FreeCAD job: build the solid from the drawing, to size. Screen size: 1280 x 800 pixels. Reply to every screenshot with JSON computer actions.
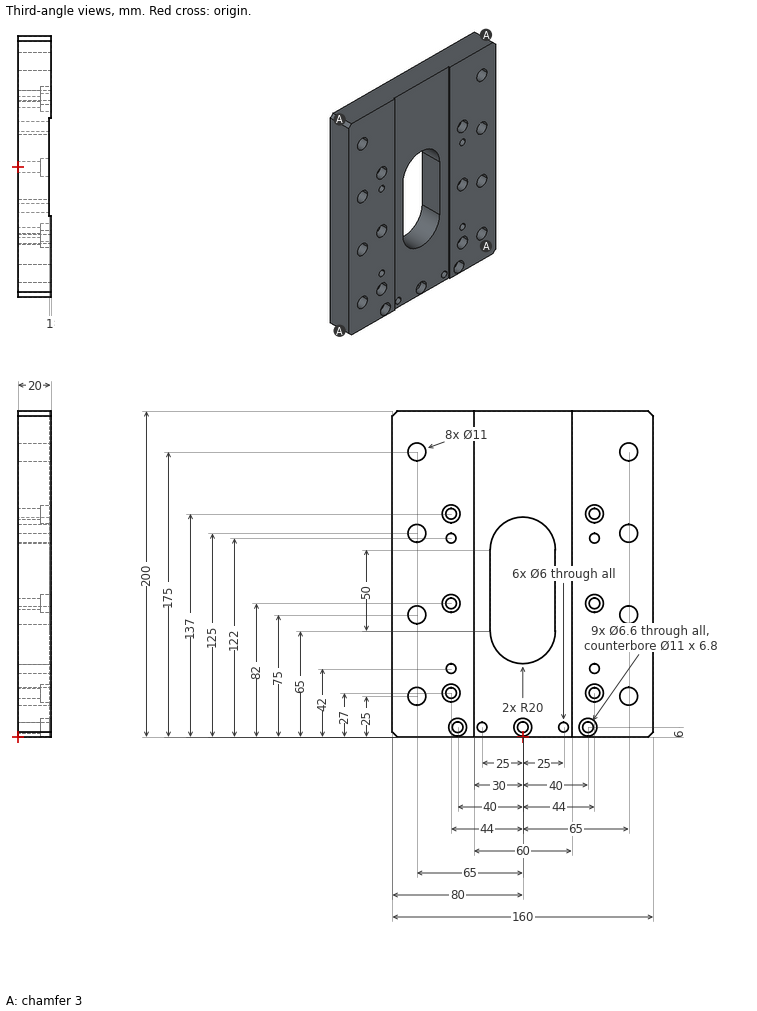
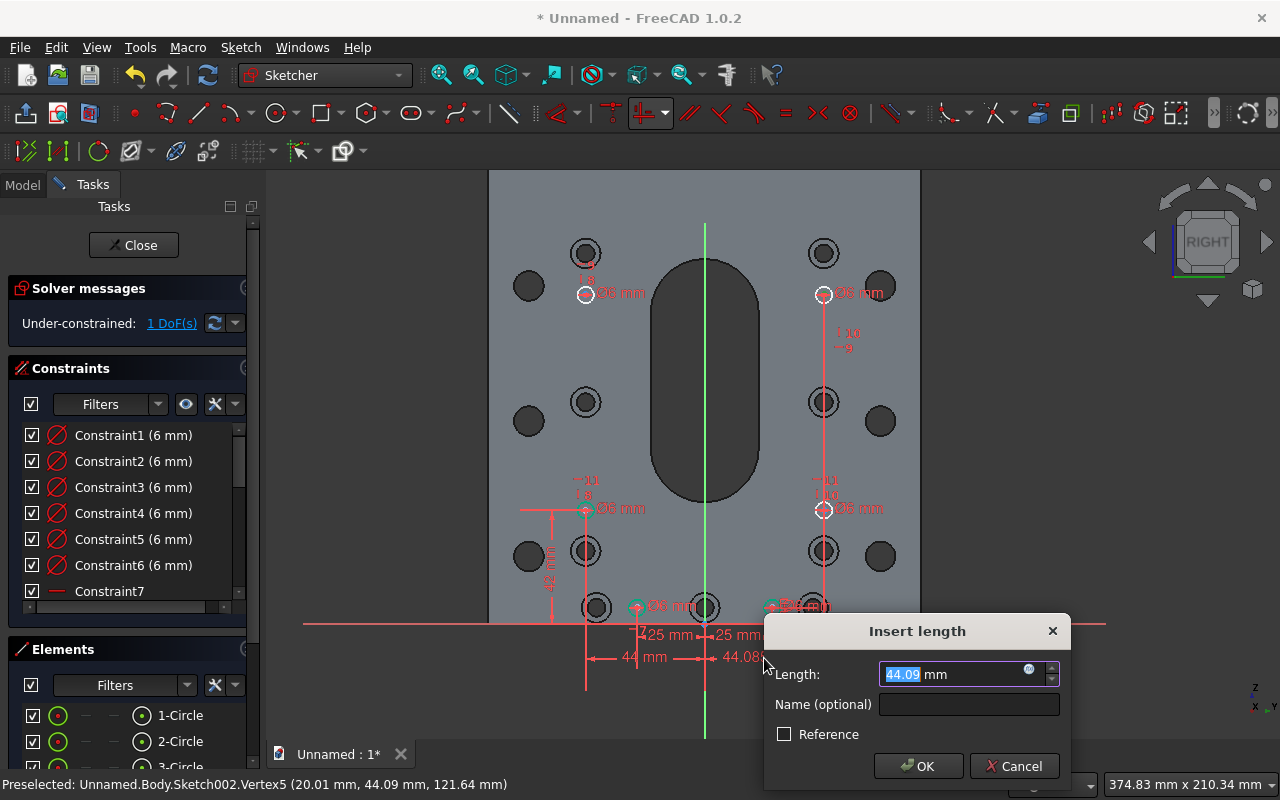
{"action": "type", "text": "44"}
{"action": "key", "text": "Return"}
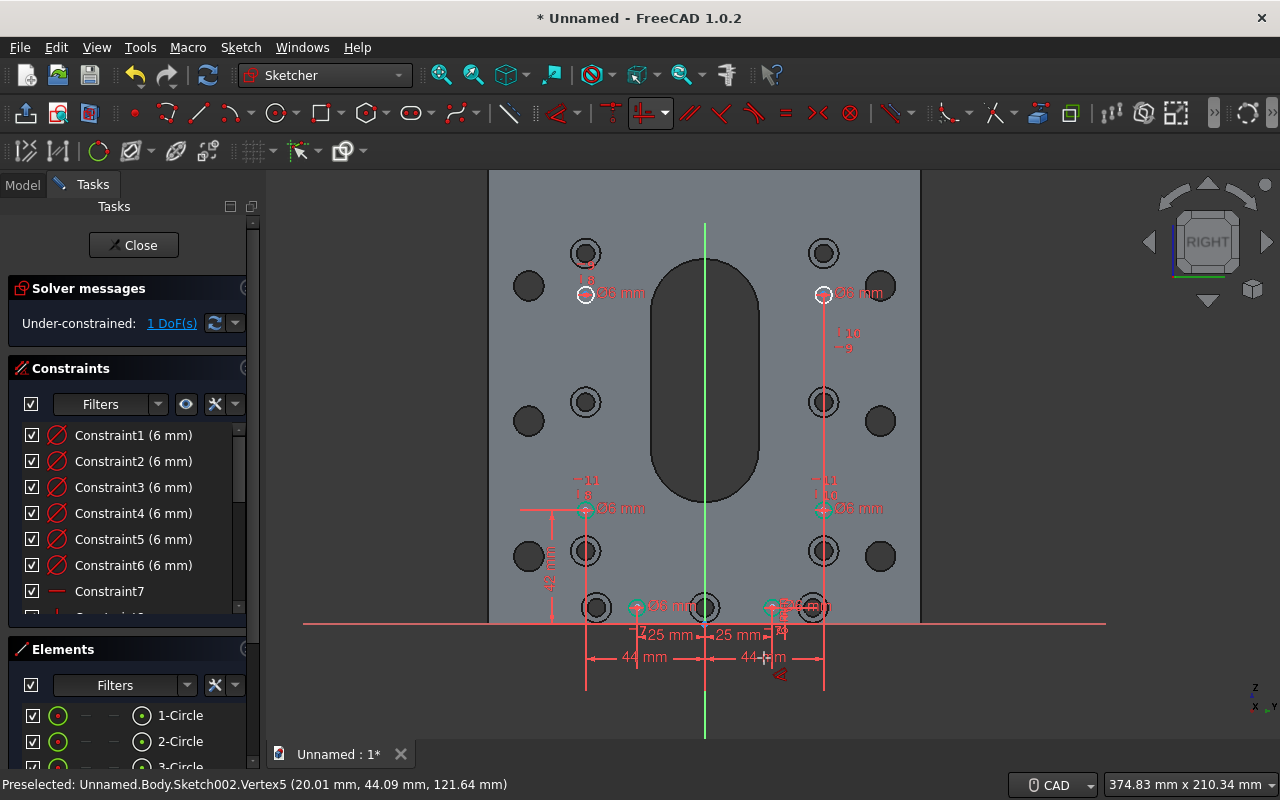
{"action": "left_click", "coordinate": [586, 295]}
{"action": "left_click", "coordinate": [552, 460]}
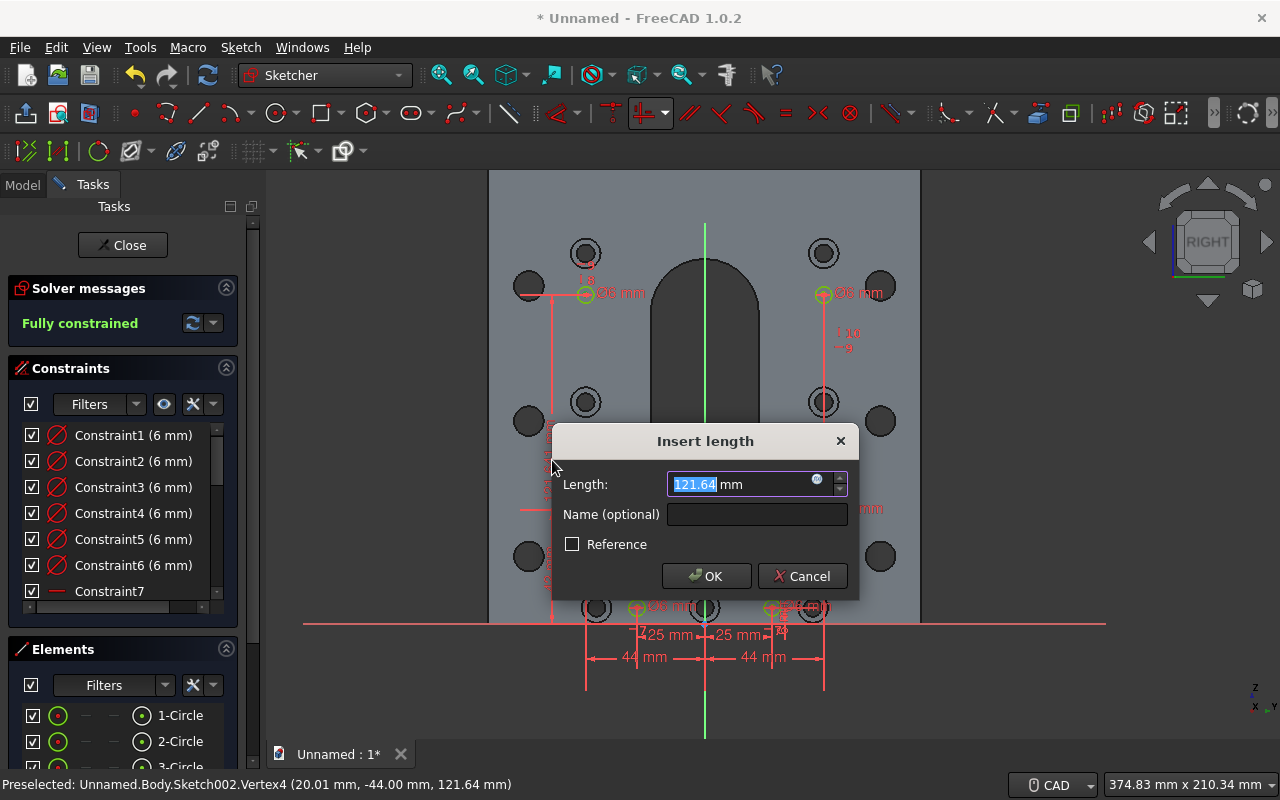
{"action": "type", "text": "122"}
{"action": "key", "text": "Return"}
{"action": "key", "text": "Escape"}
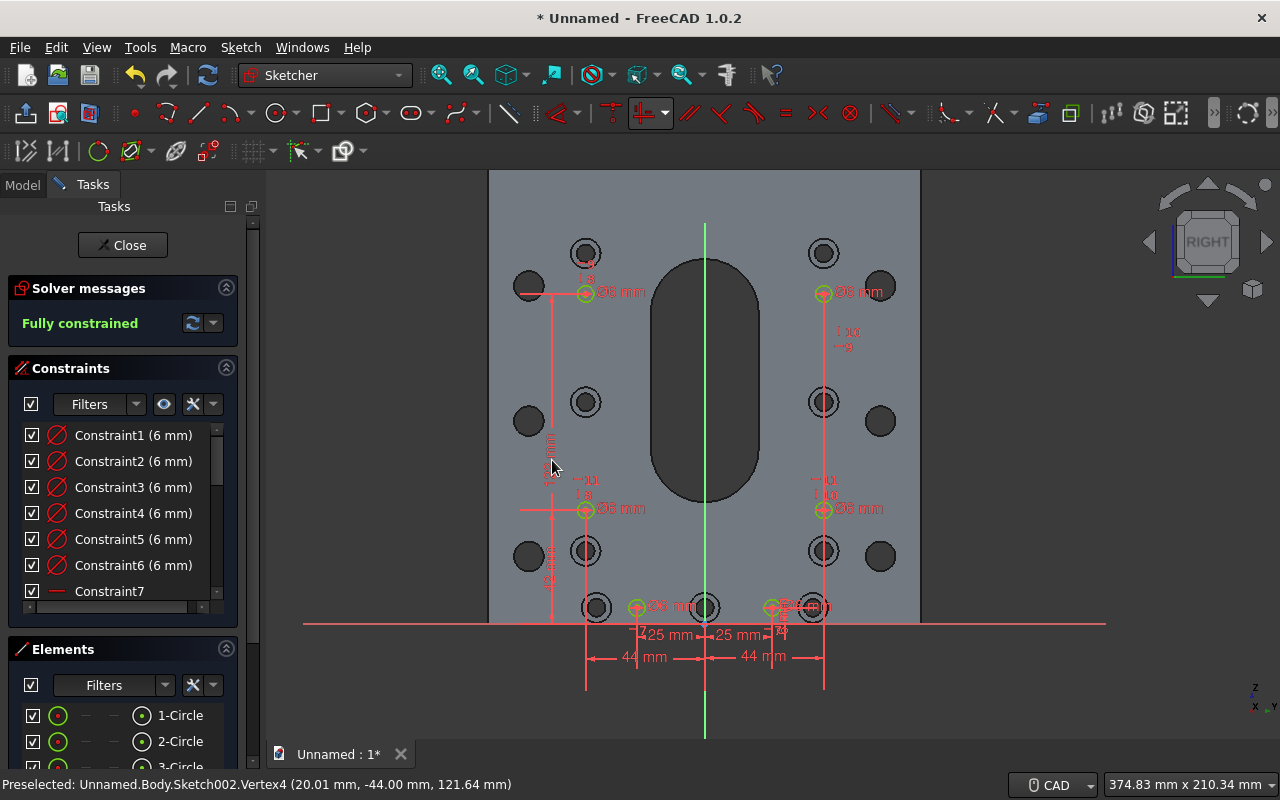
{"action": "left_click", "coordinate": [123, 245]}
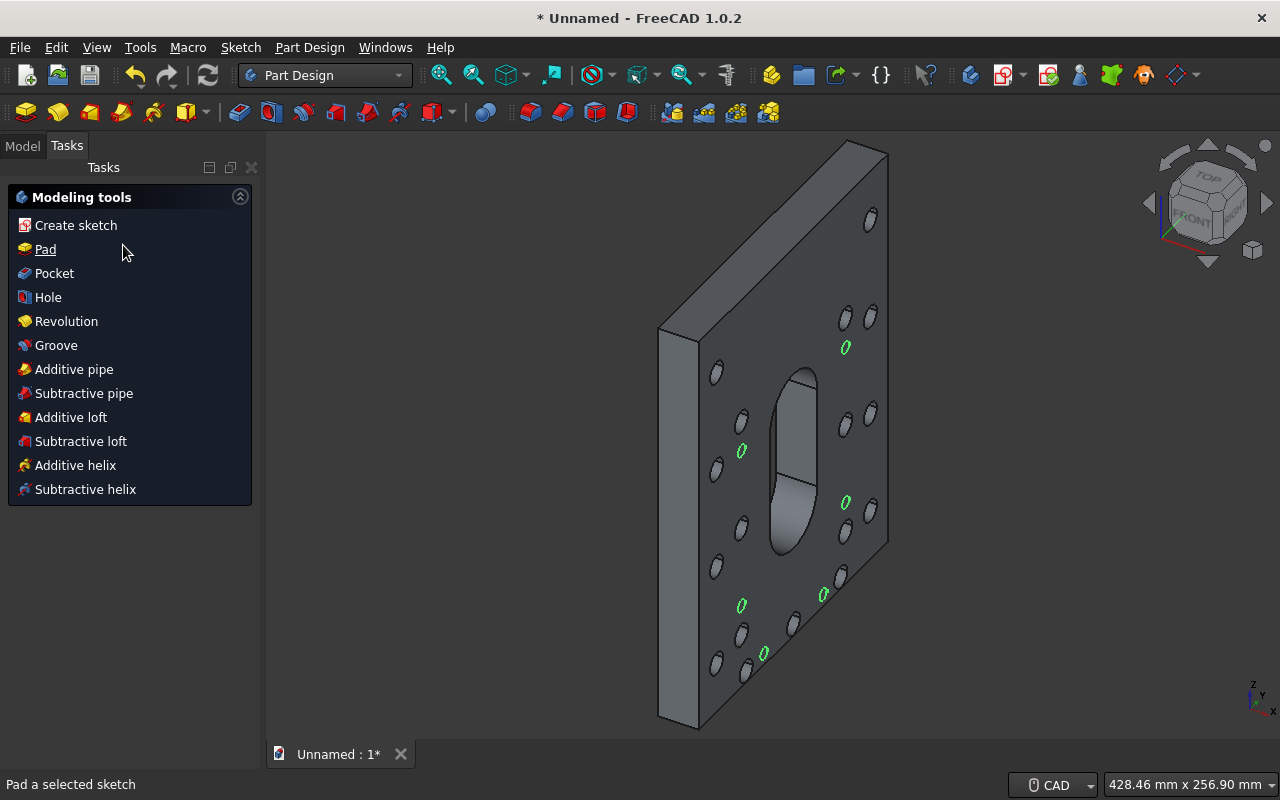
{"action": "left_click", "coordinate": [272, 112]}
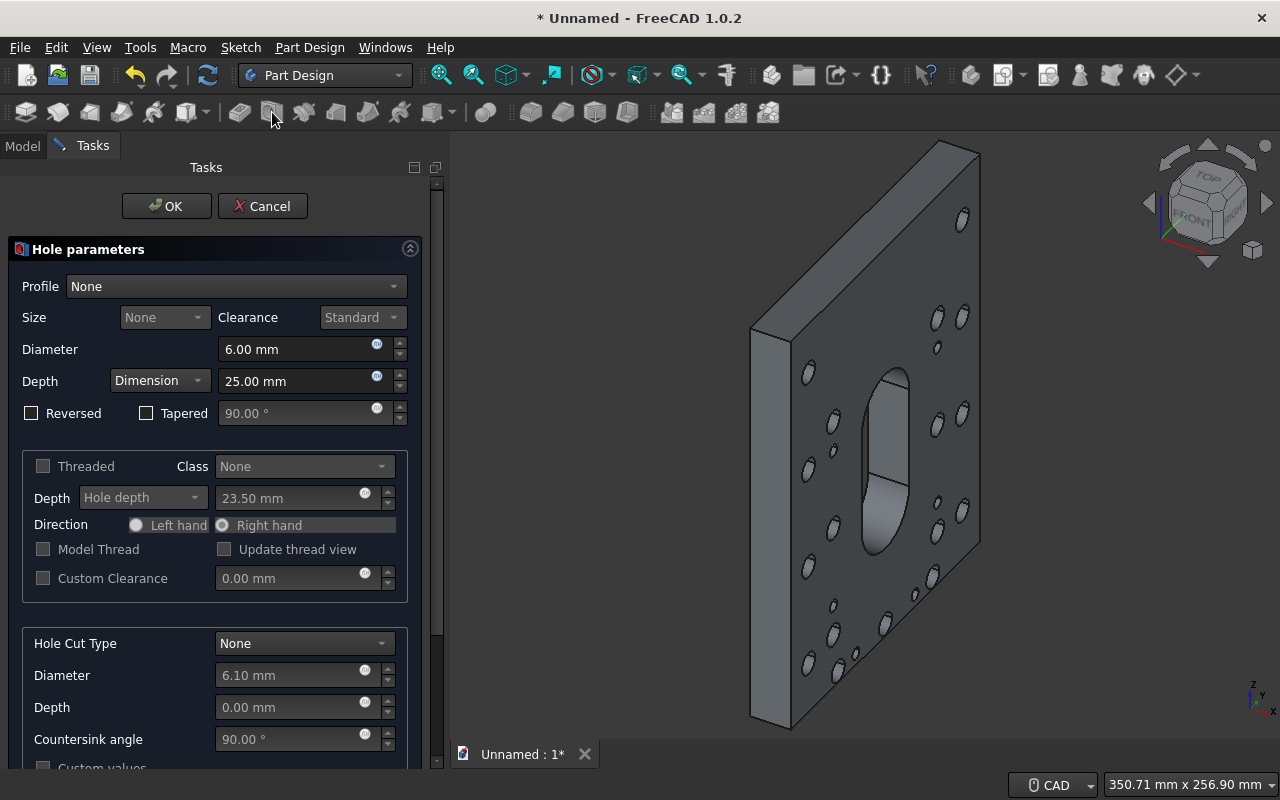
{"action": "triple_click", "coordinate": [305, 349]}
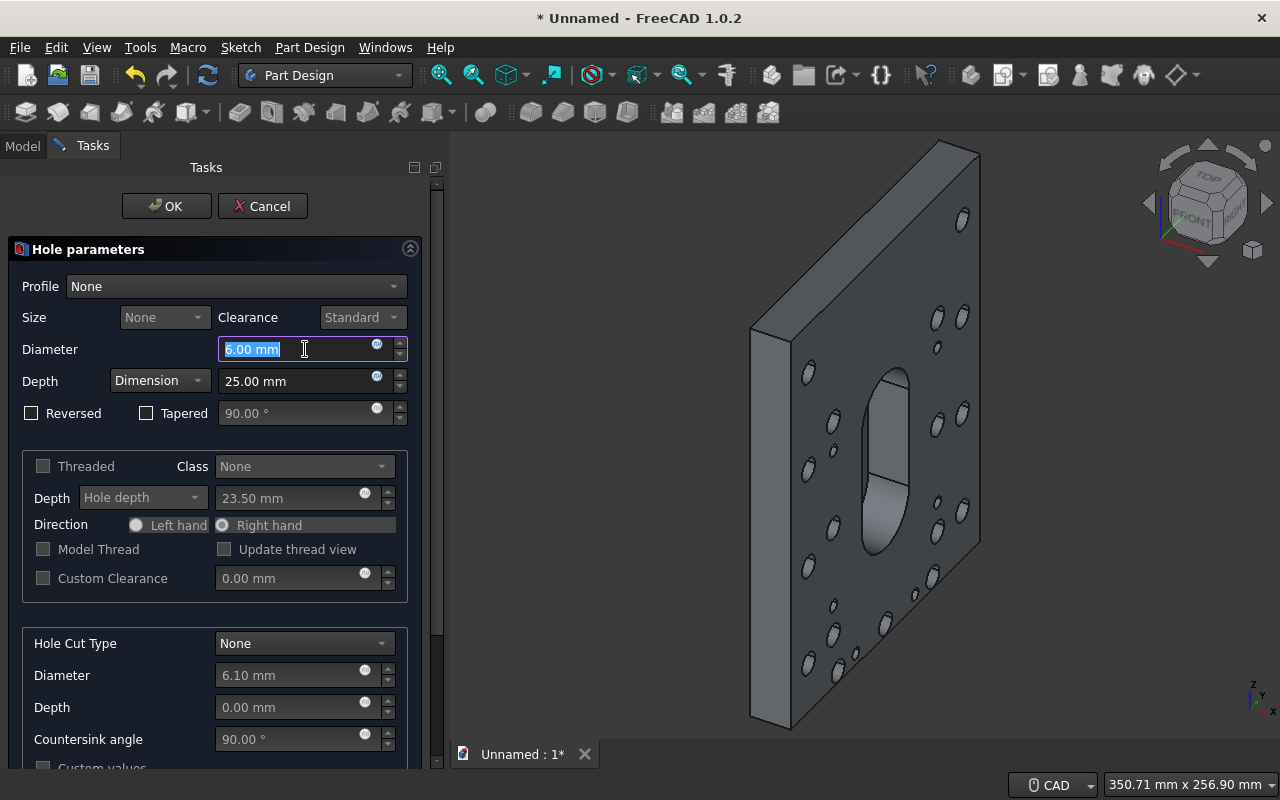
{"action": "type", "text": "6"}
{"action": "key", "text": "Tab"}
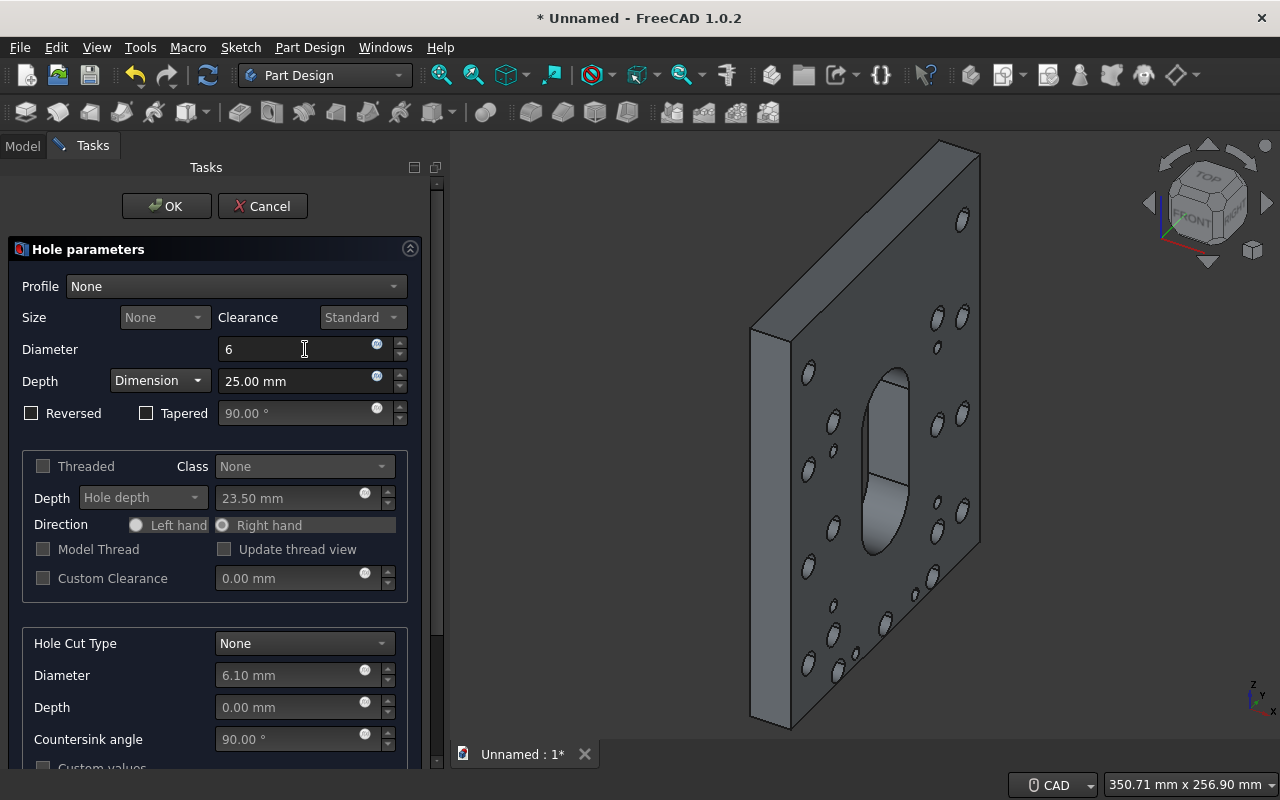
{"action": "left_click", "coordinate": [161, 380]}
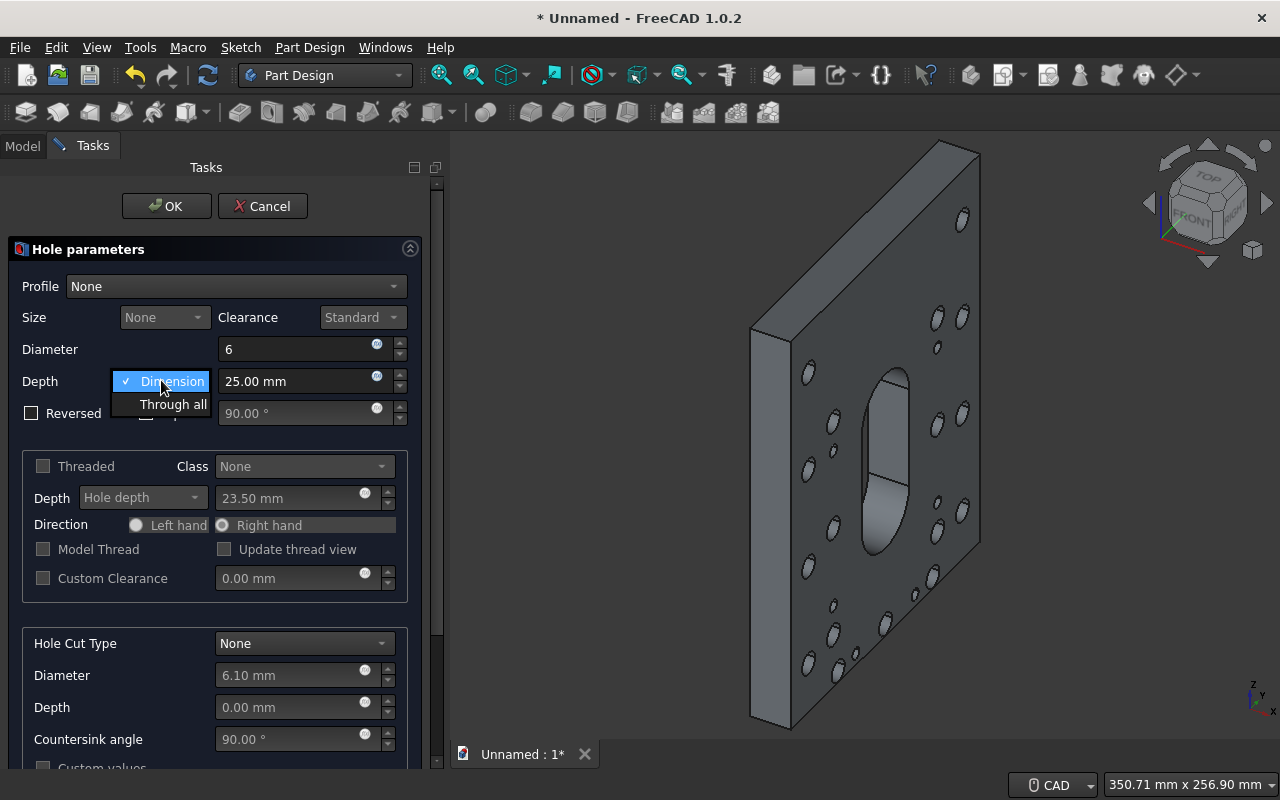
{"action": "left_click", "coordinate": [160, 404]}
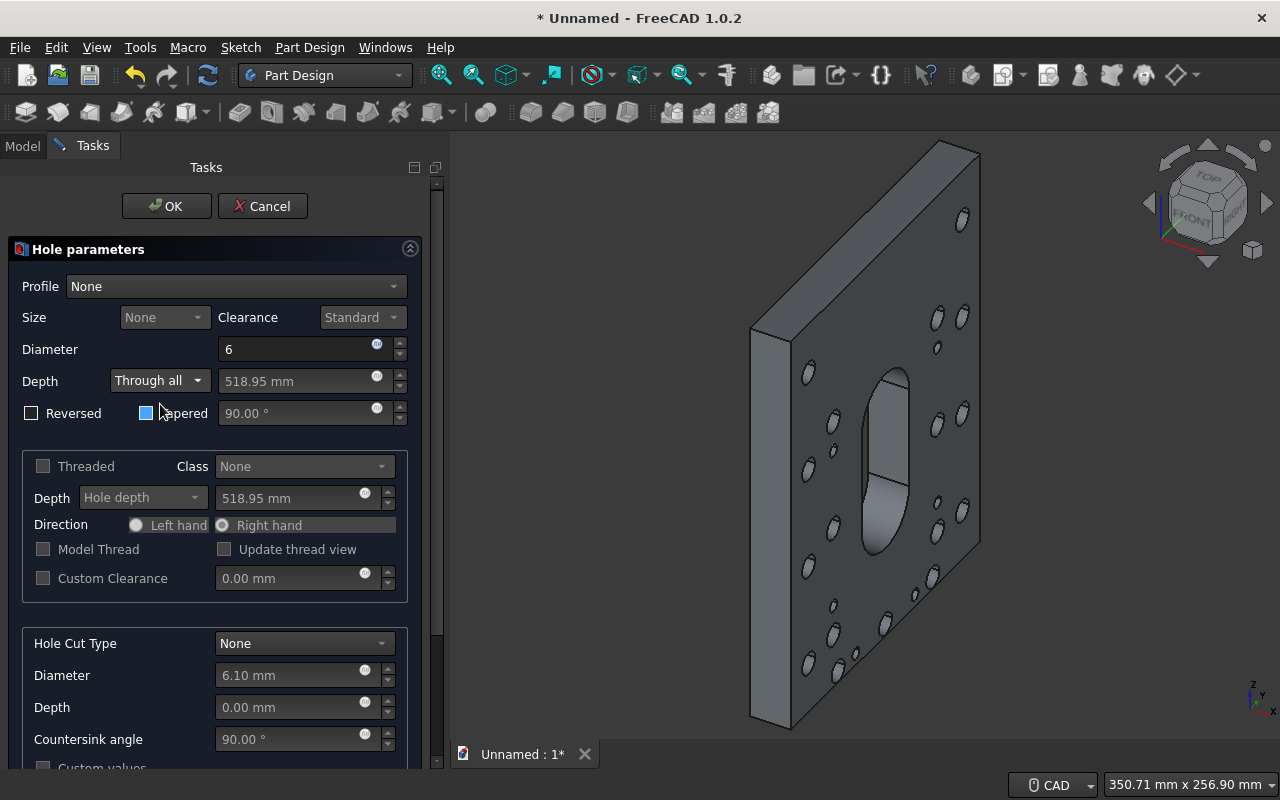
{"action": "left_click", "coordinate": [167, 206]}